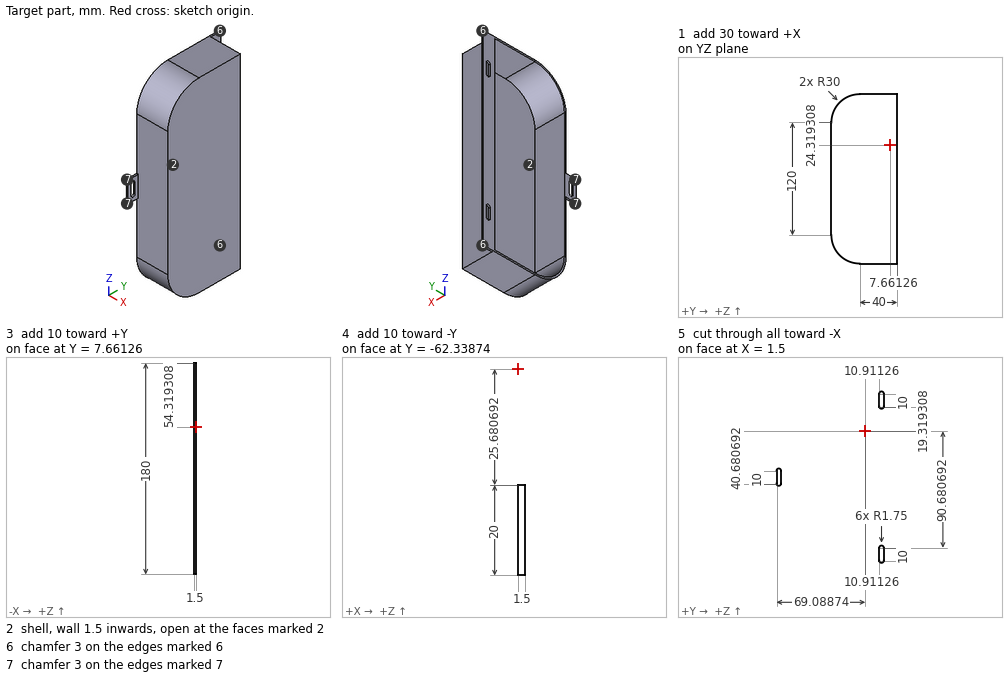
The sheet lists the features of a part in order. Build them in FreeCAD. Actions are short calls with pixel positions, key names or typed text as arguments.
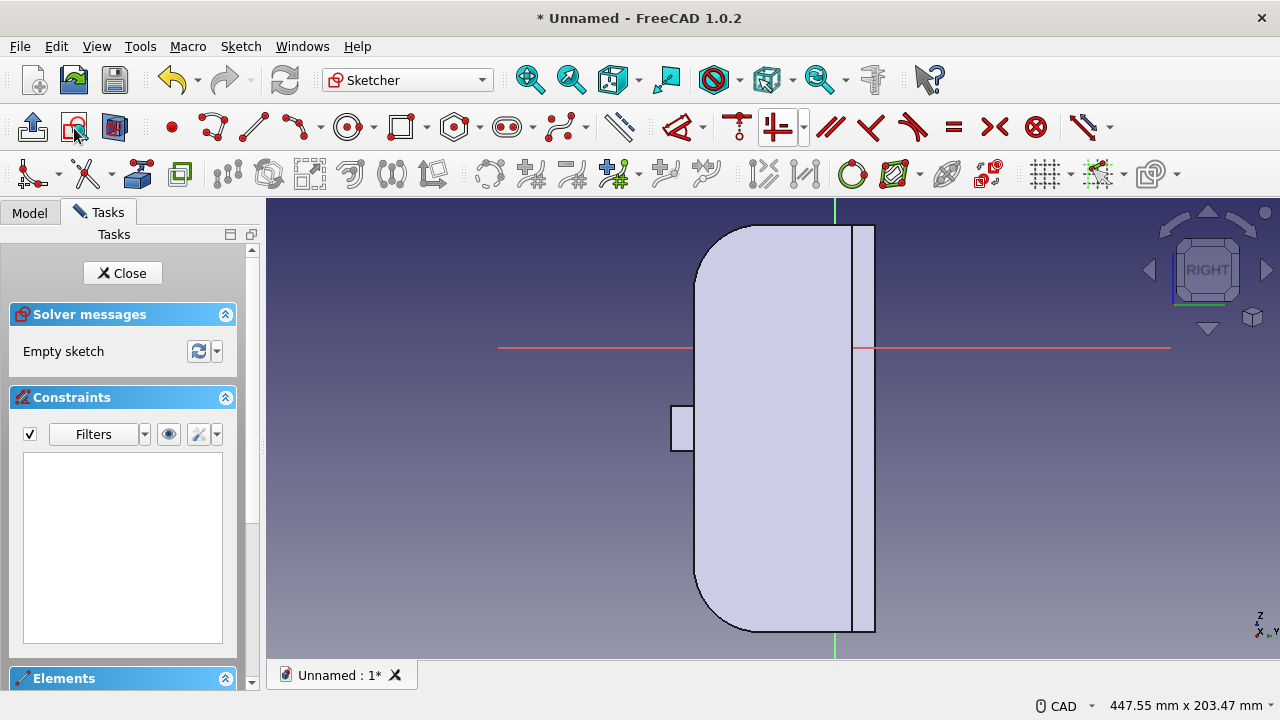
click(506, 128)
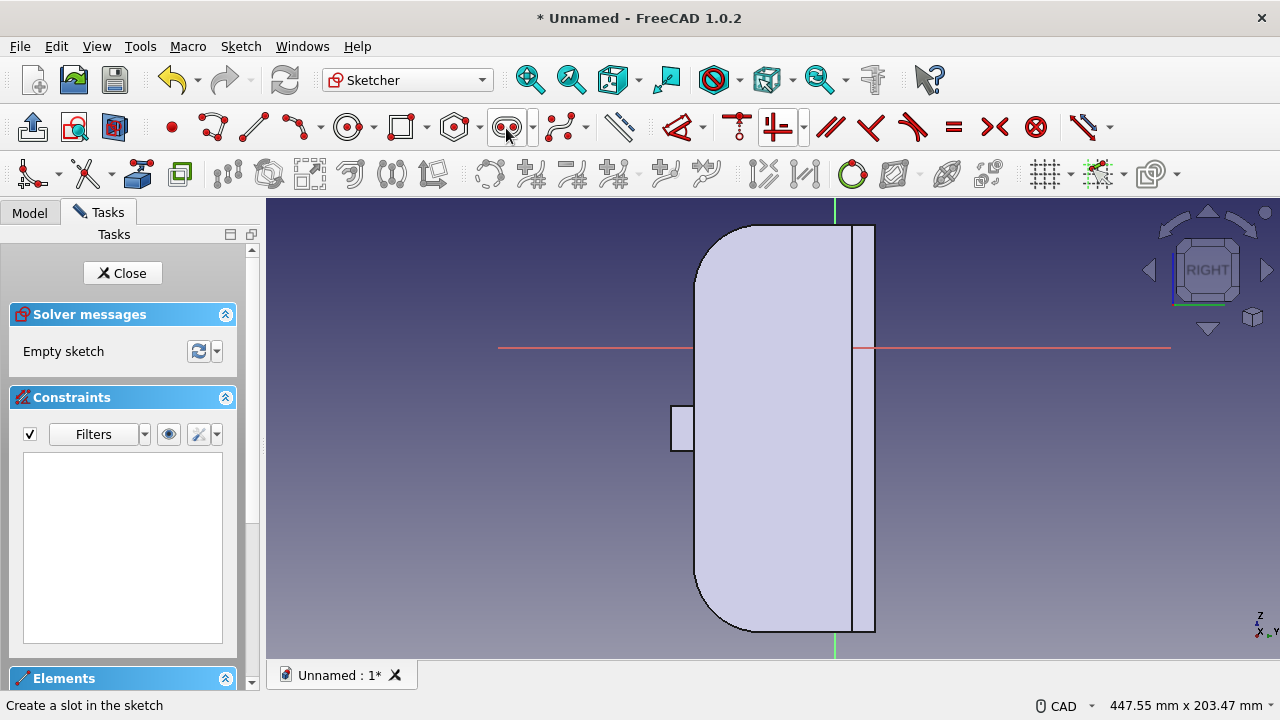
scroll(864, 304, up, 9)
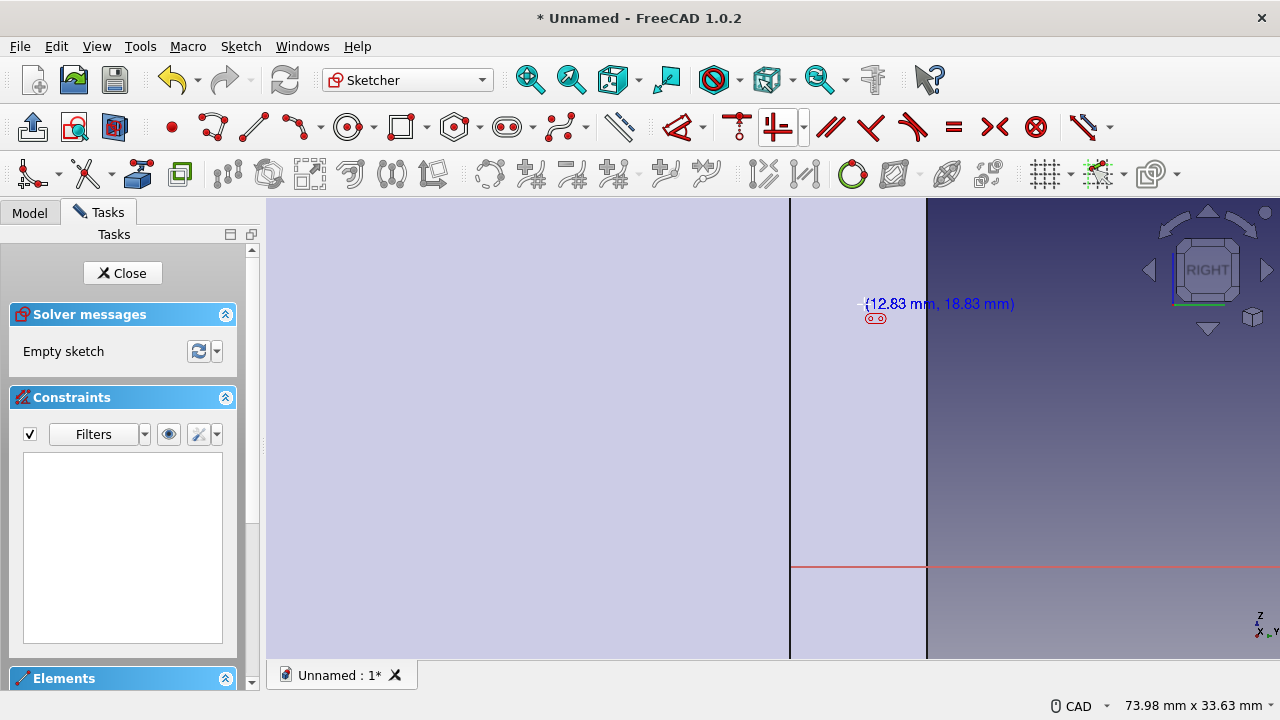
scroll(783, 304, down, 9)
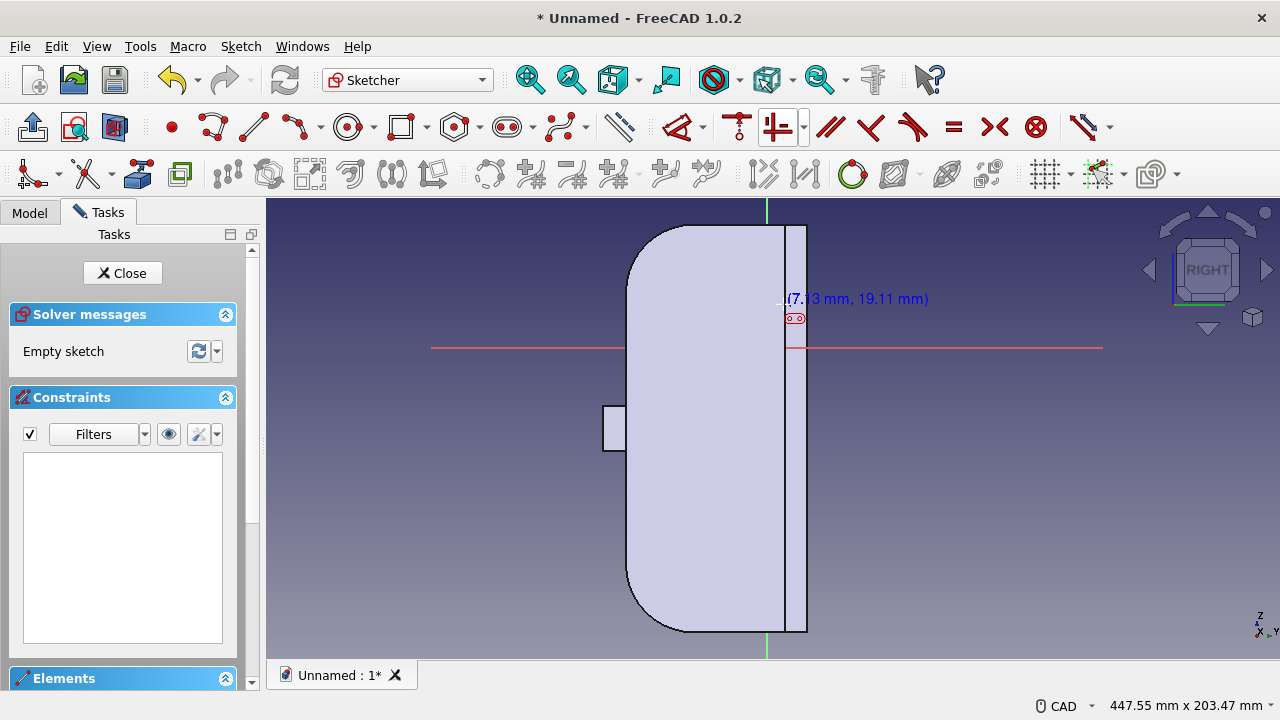
click(796, 304)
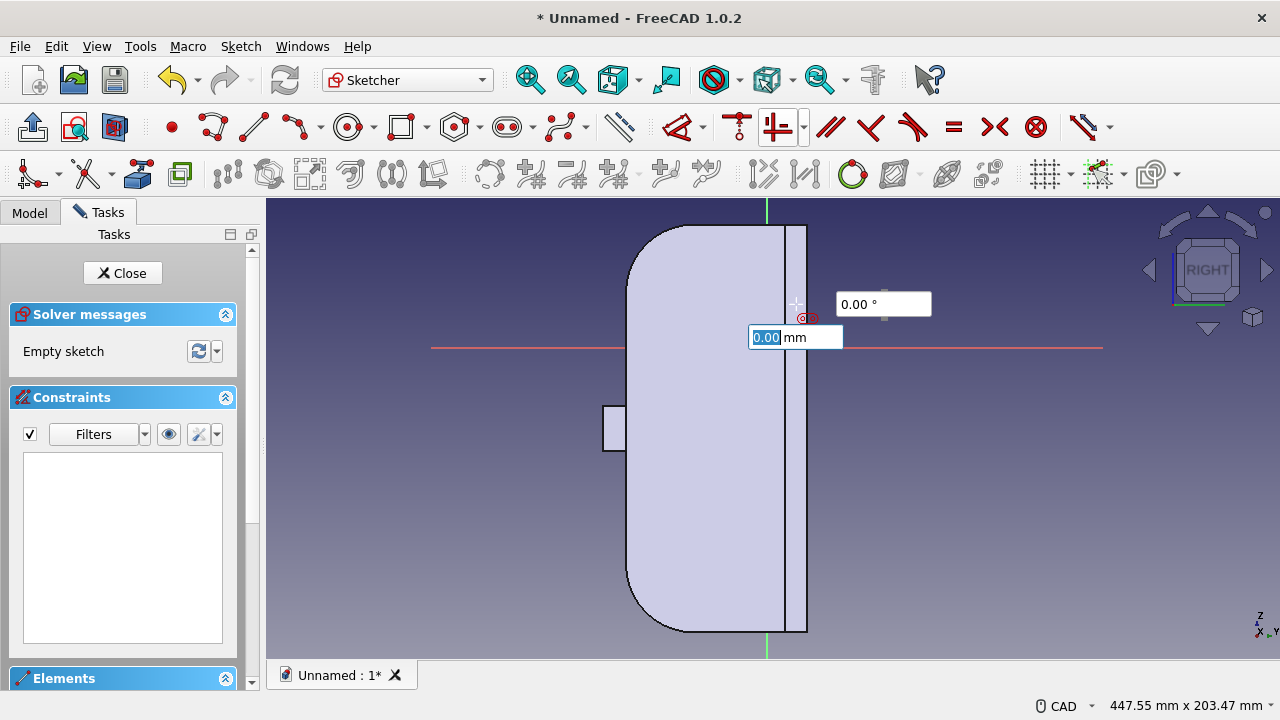
click(796, 281)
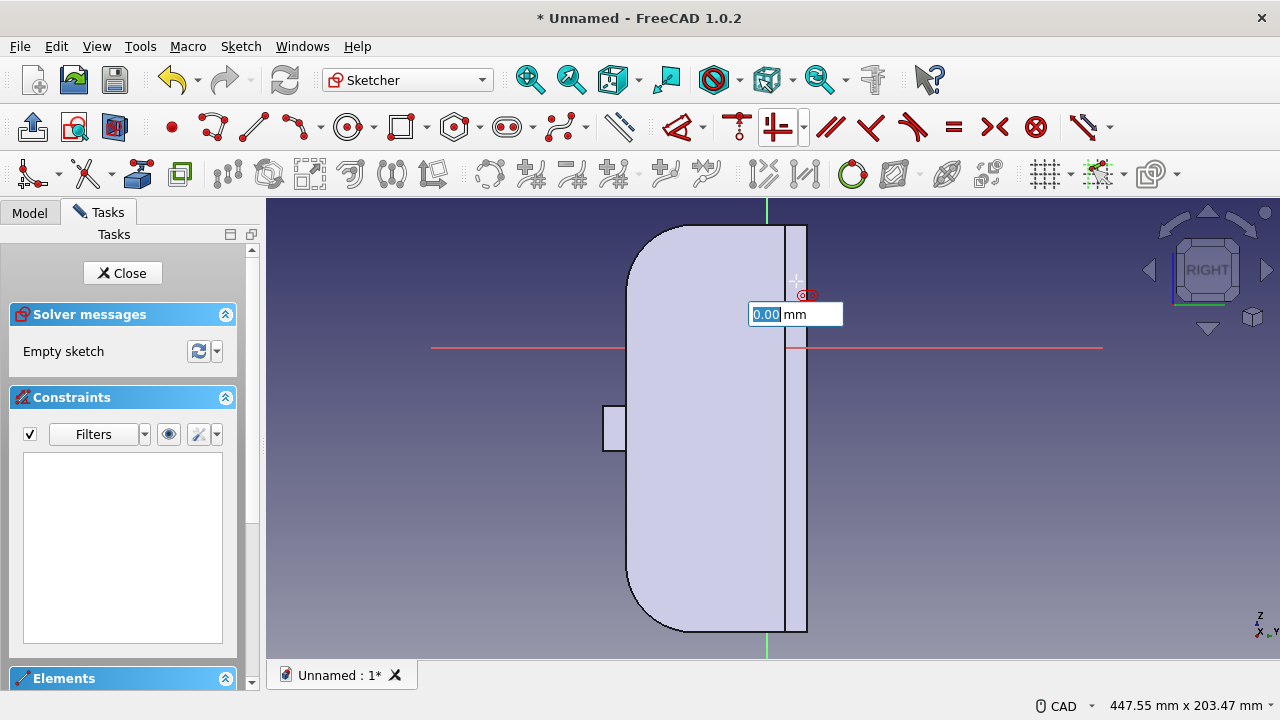
scroll(800, 293, up, 7)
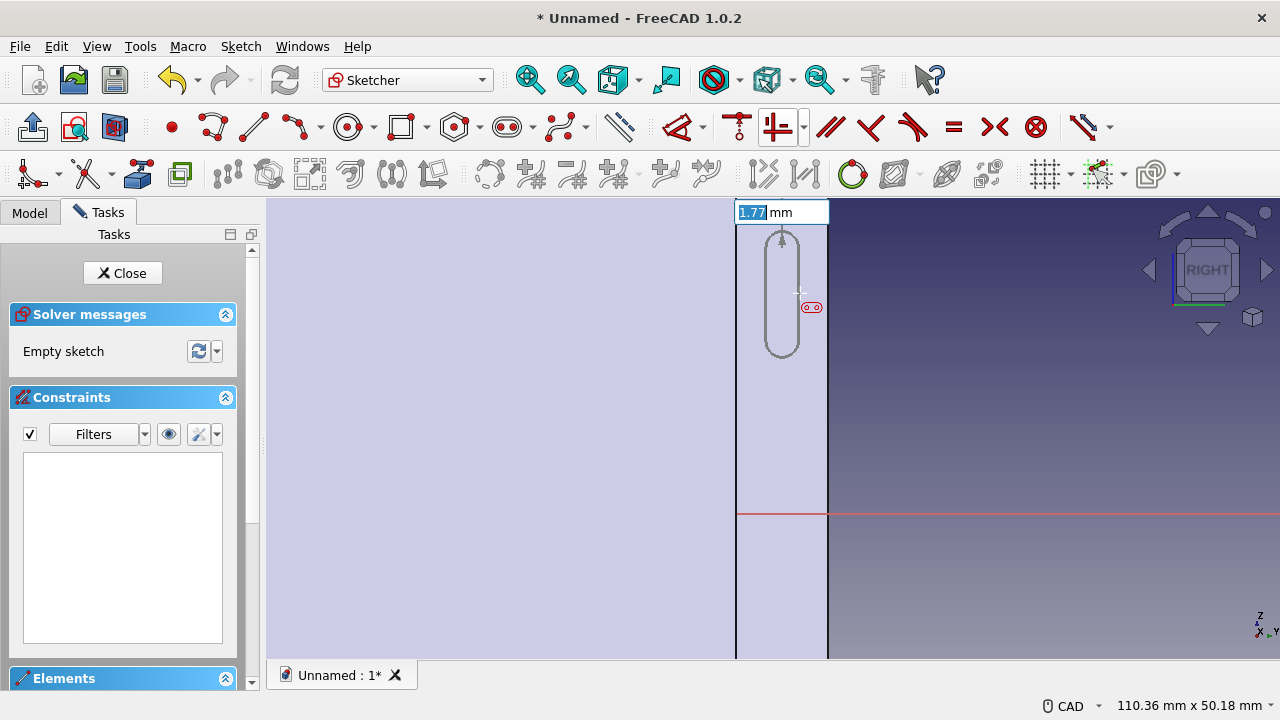
click(798, 291)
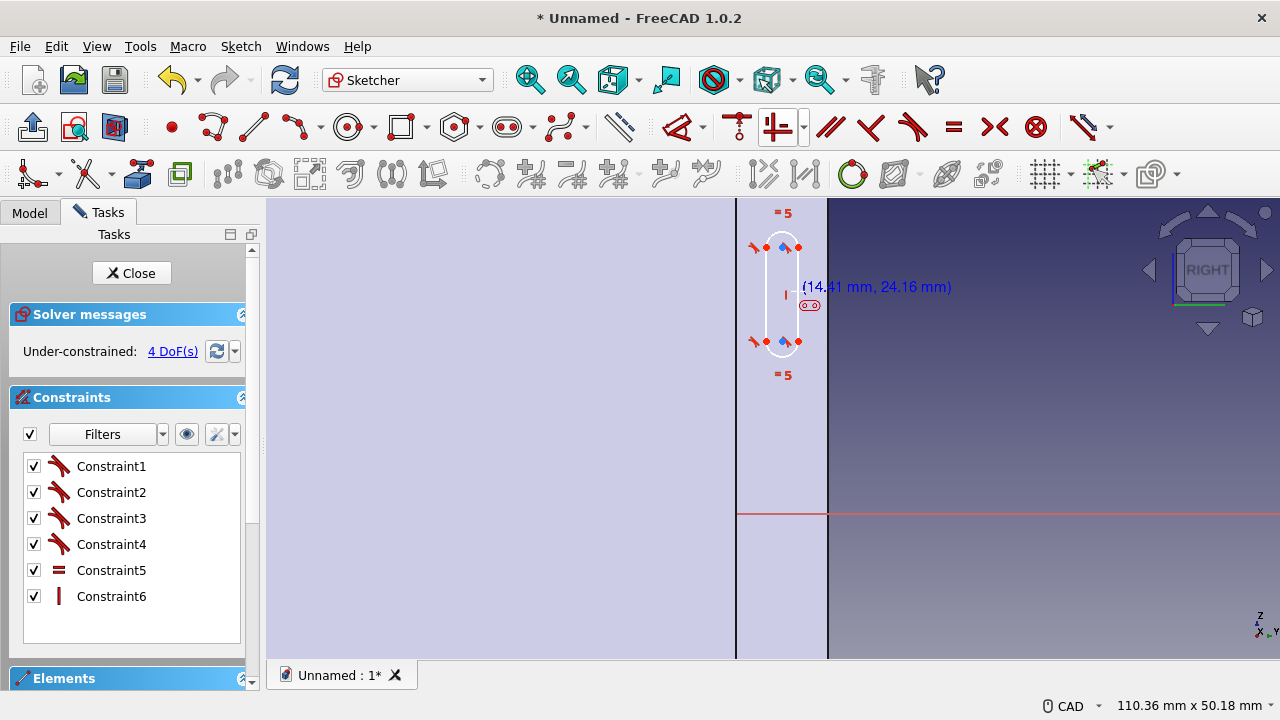
scroll(799, 293, down, 7)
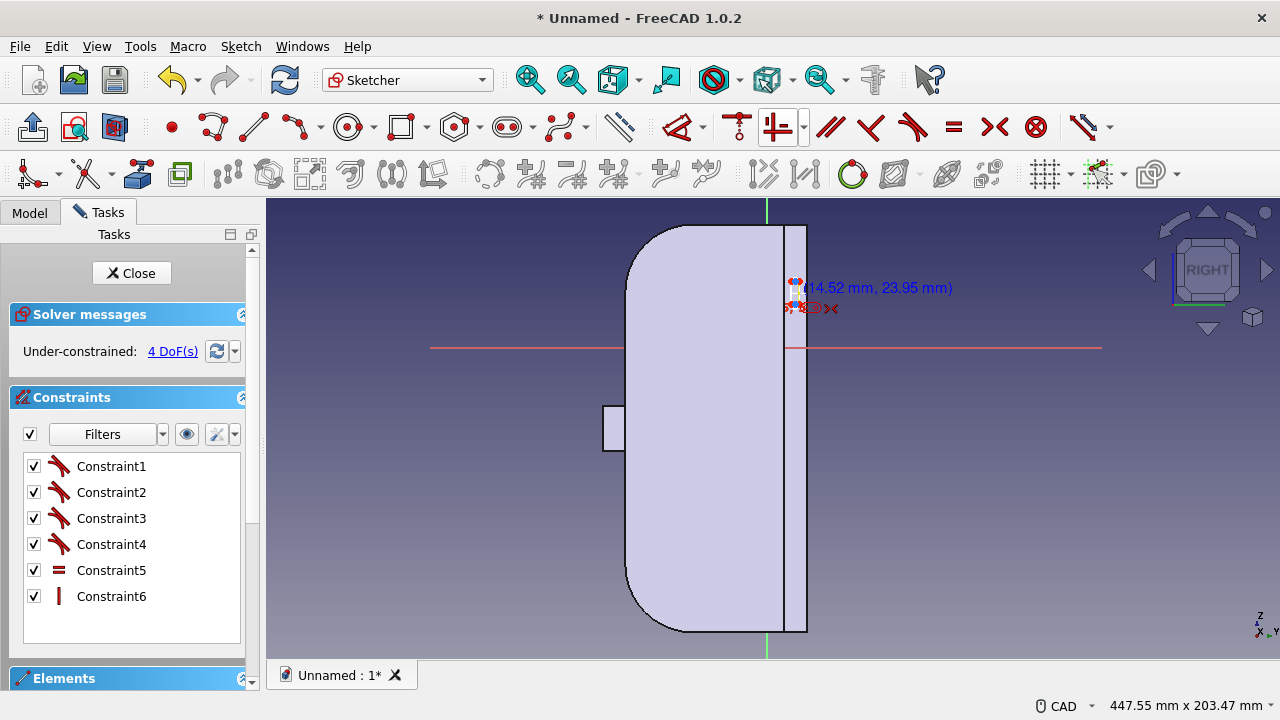
scroll(795, 576, up, 9)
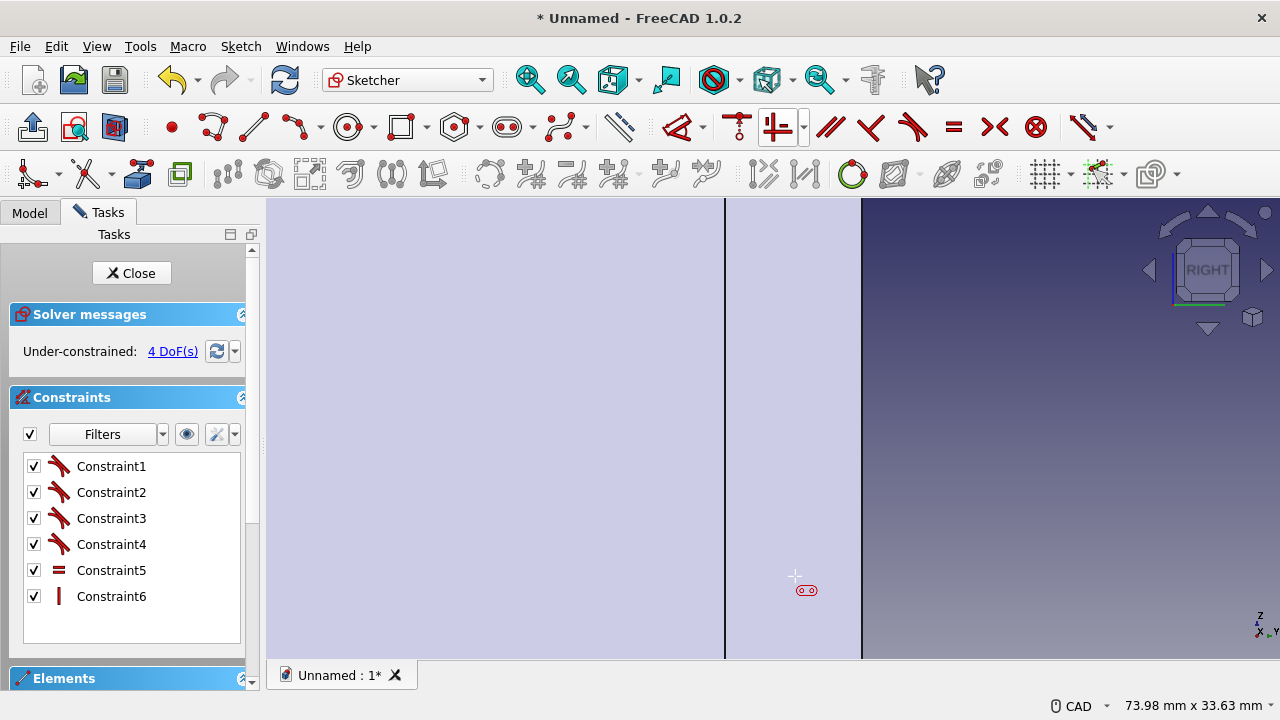
scroll(795, 577, down, 9)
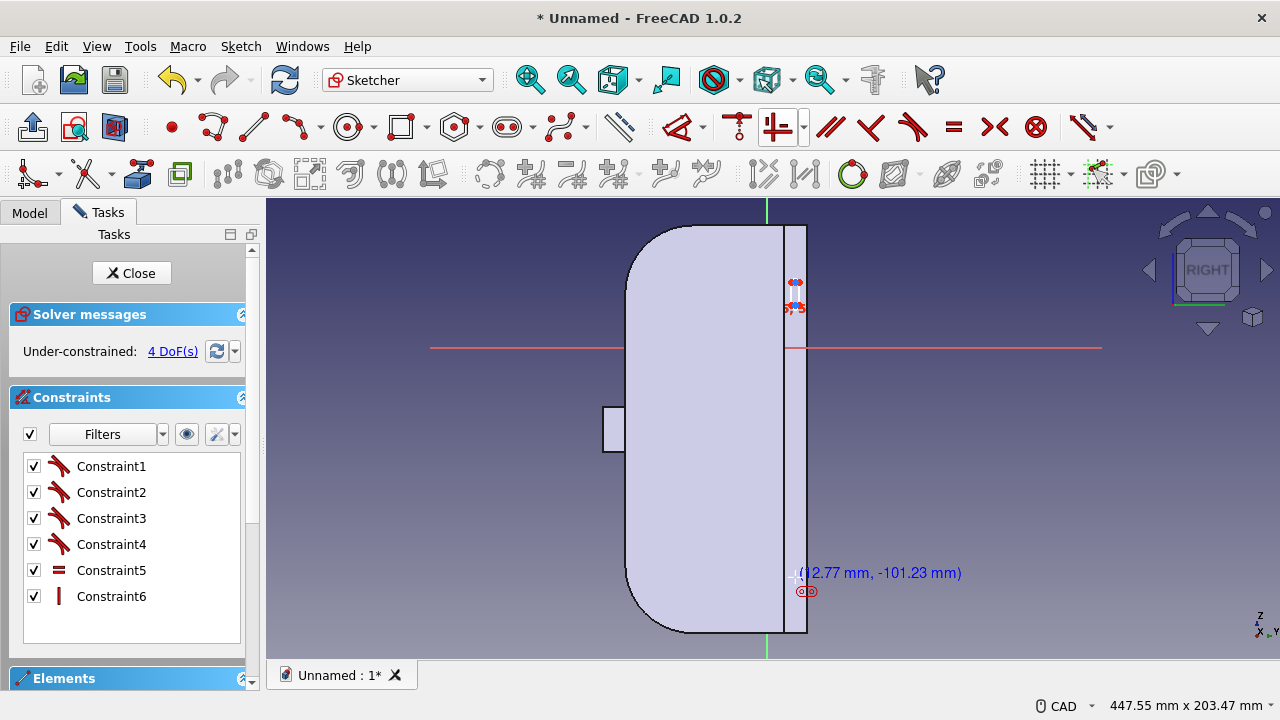
click(795, 577)